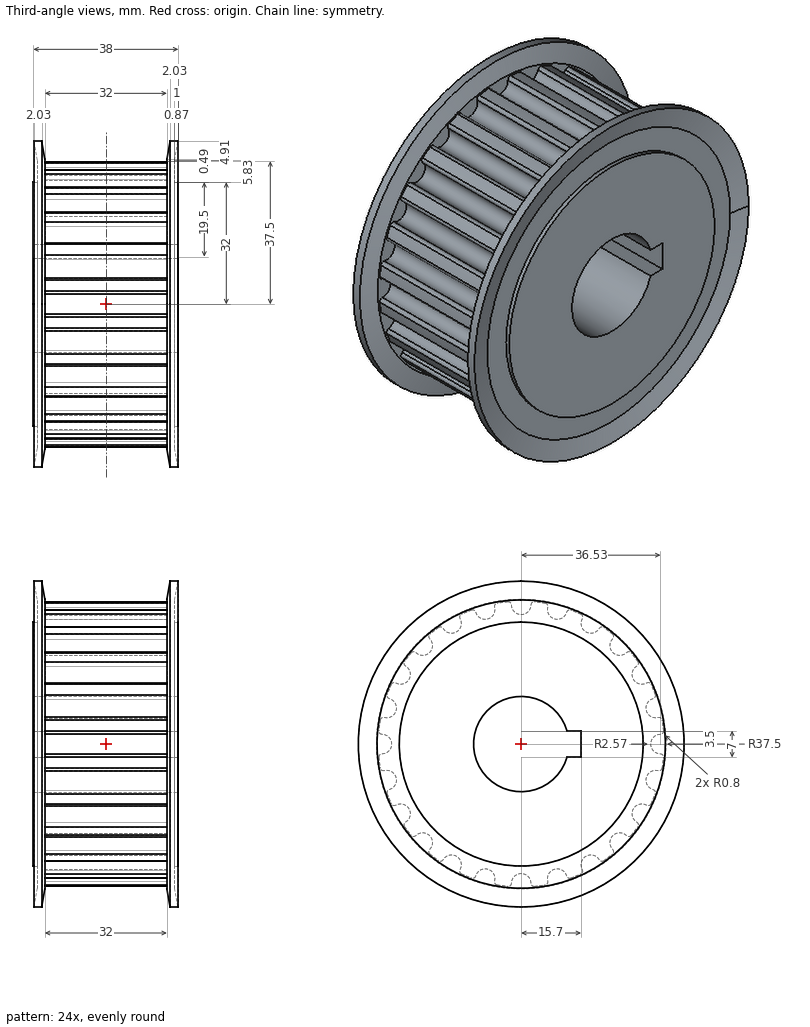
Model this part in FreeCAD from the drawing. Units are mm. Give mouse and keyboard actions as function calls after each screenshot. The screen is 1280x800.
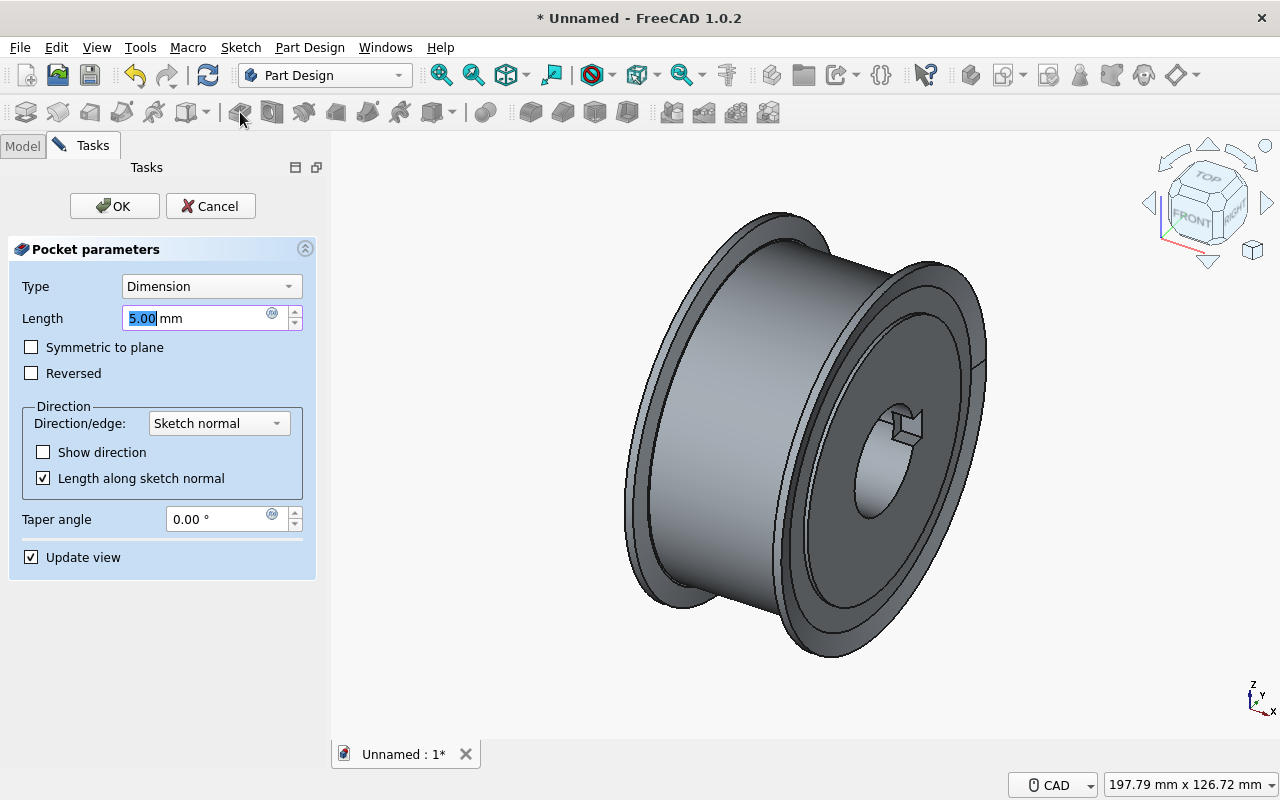
click(212, 286)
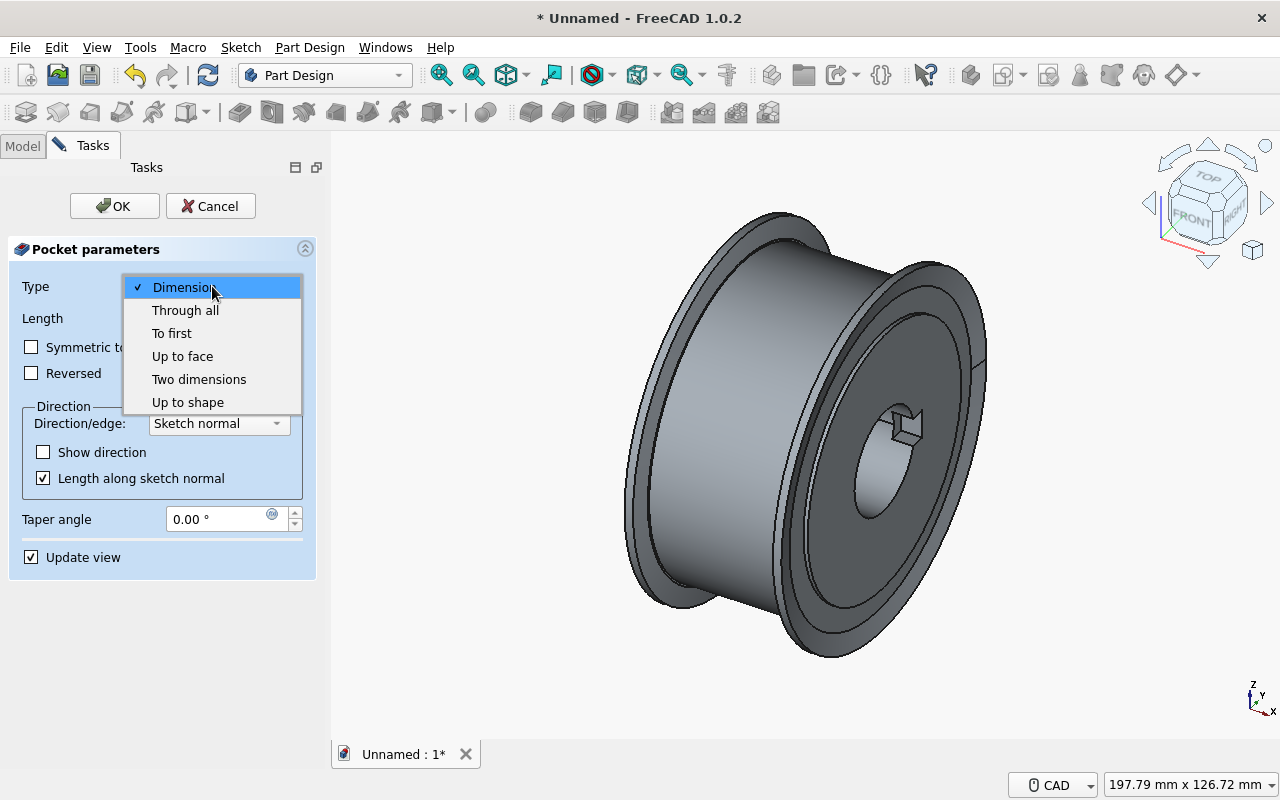
click(212, 310)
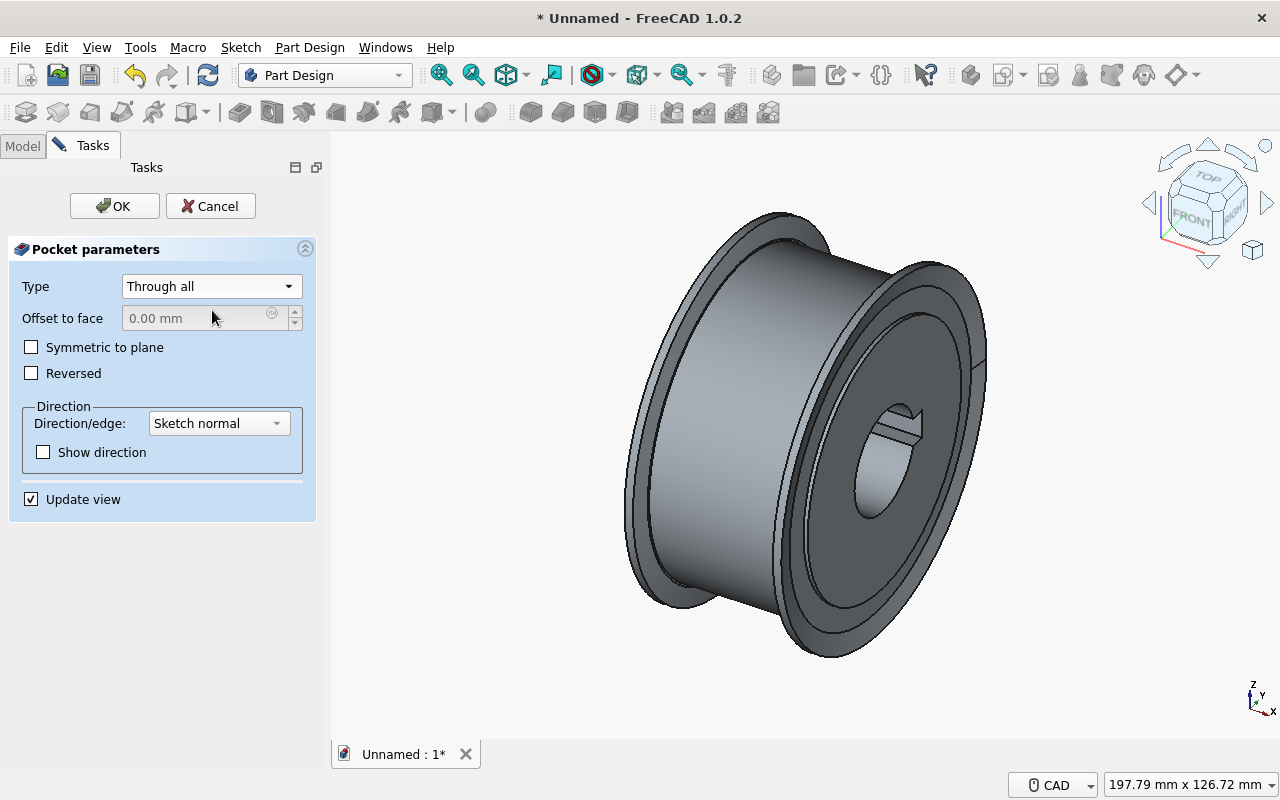
click(115, 206)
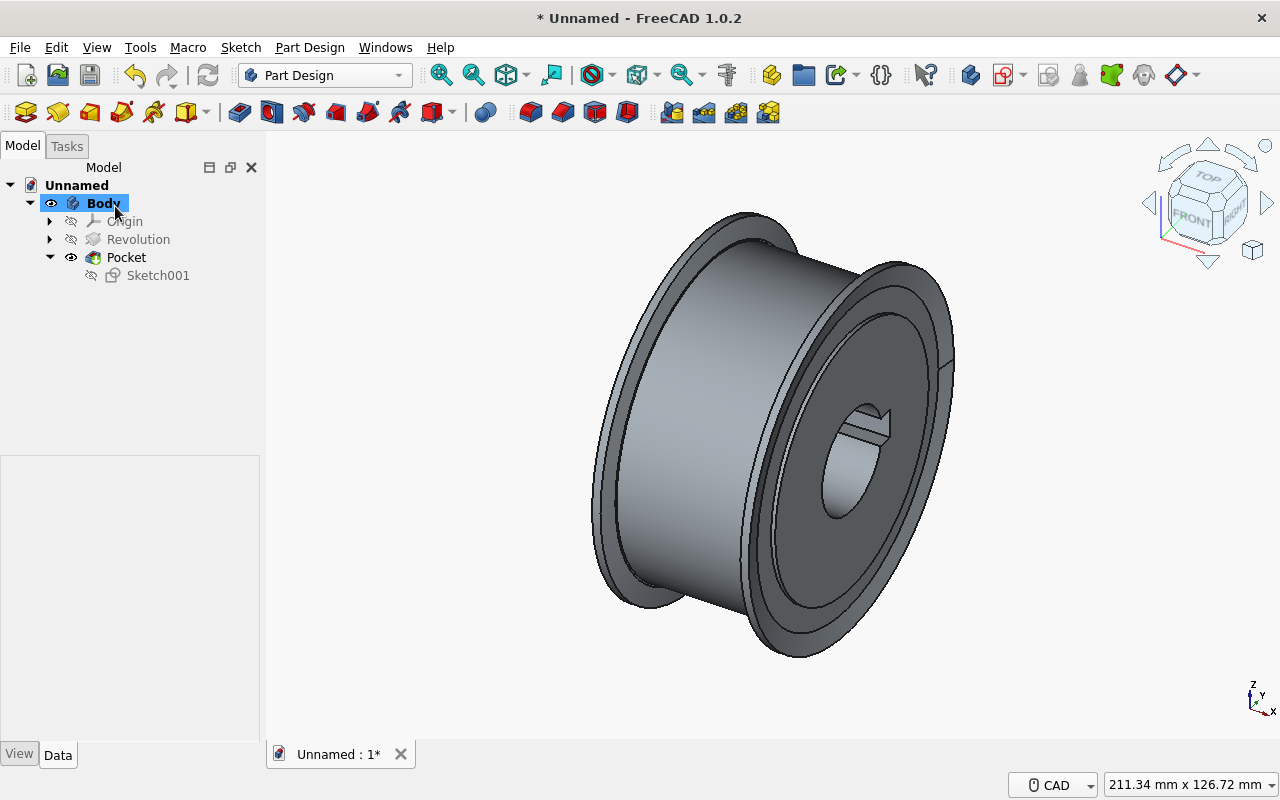
click(50, 221)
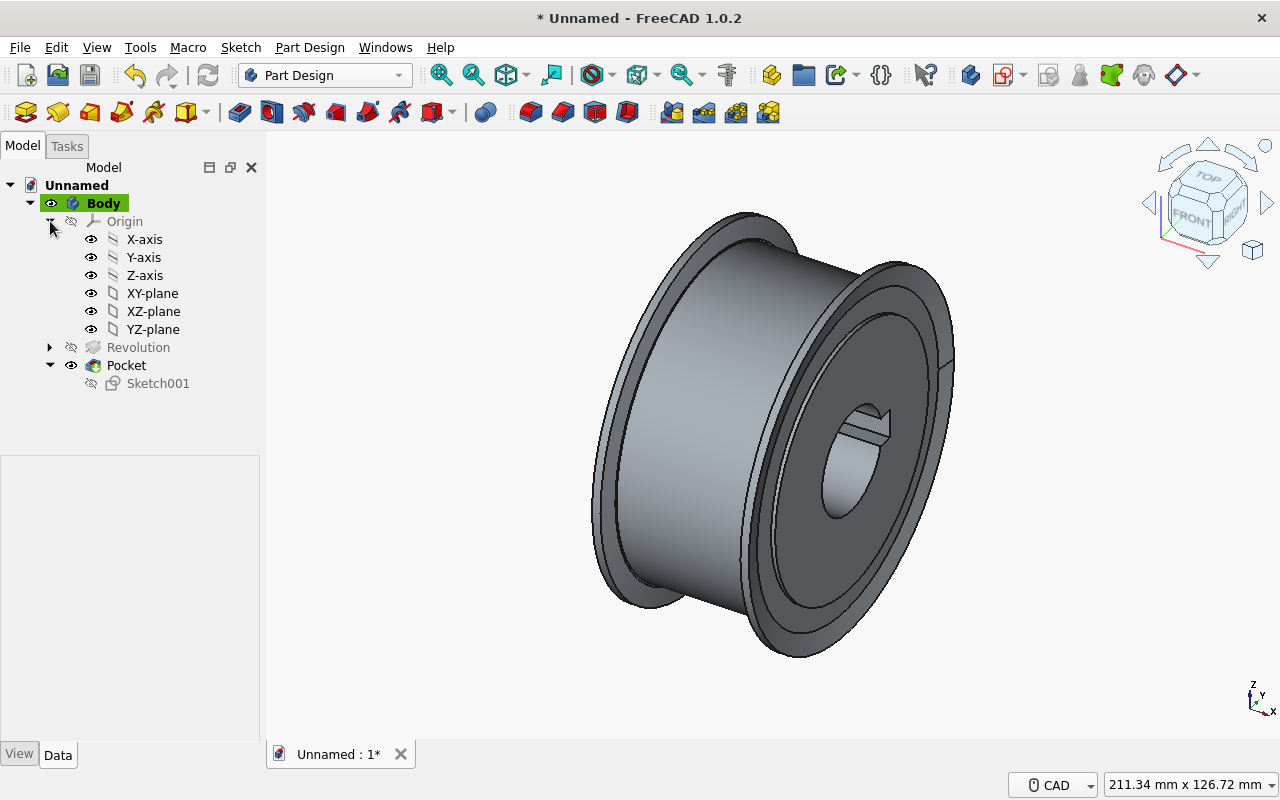
click(136, 329)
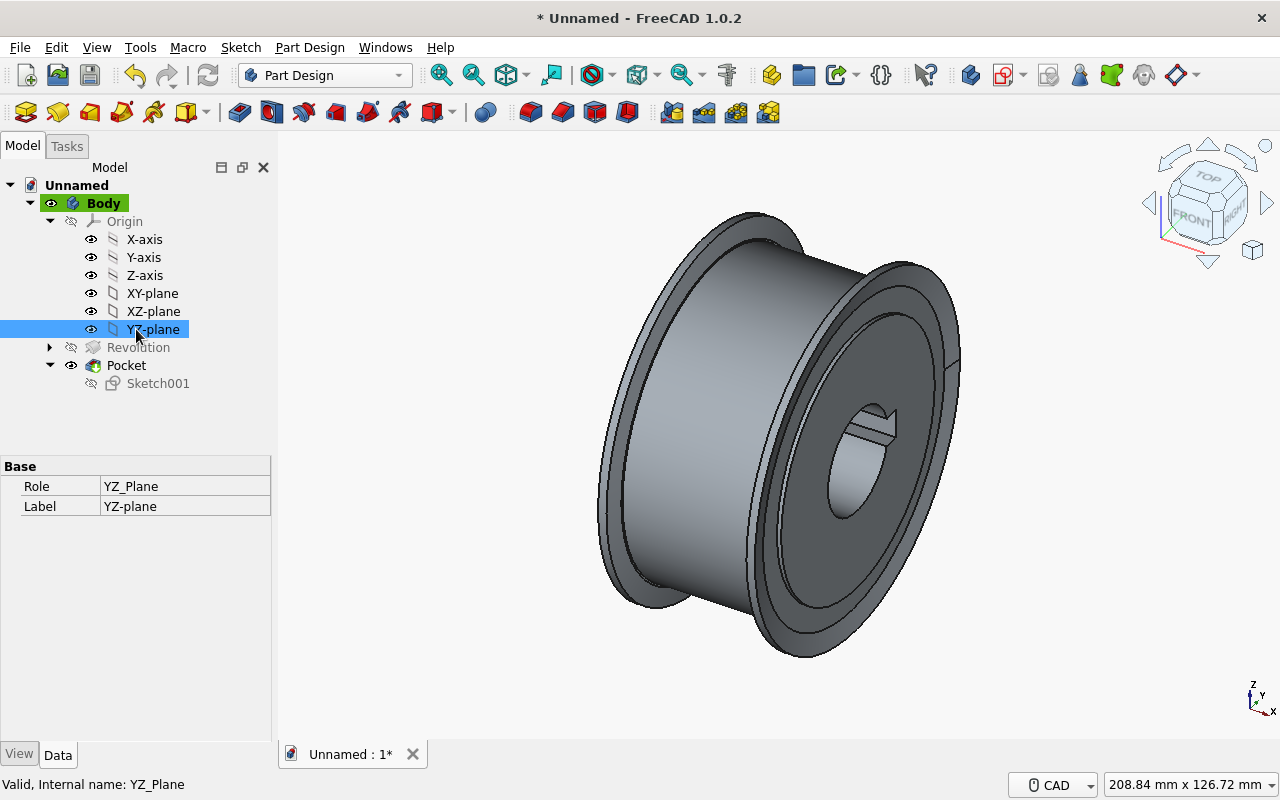
click(1176, 76)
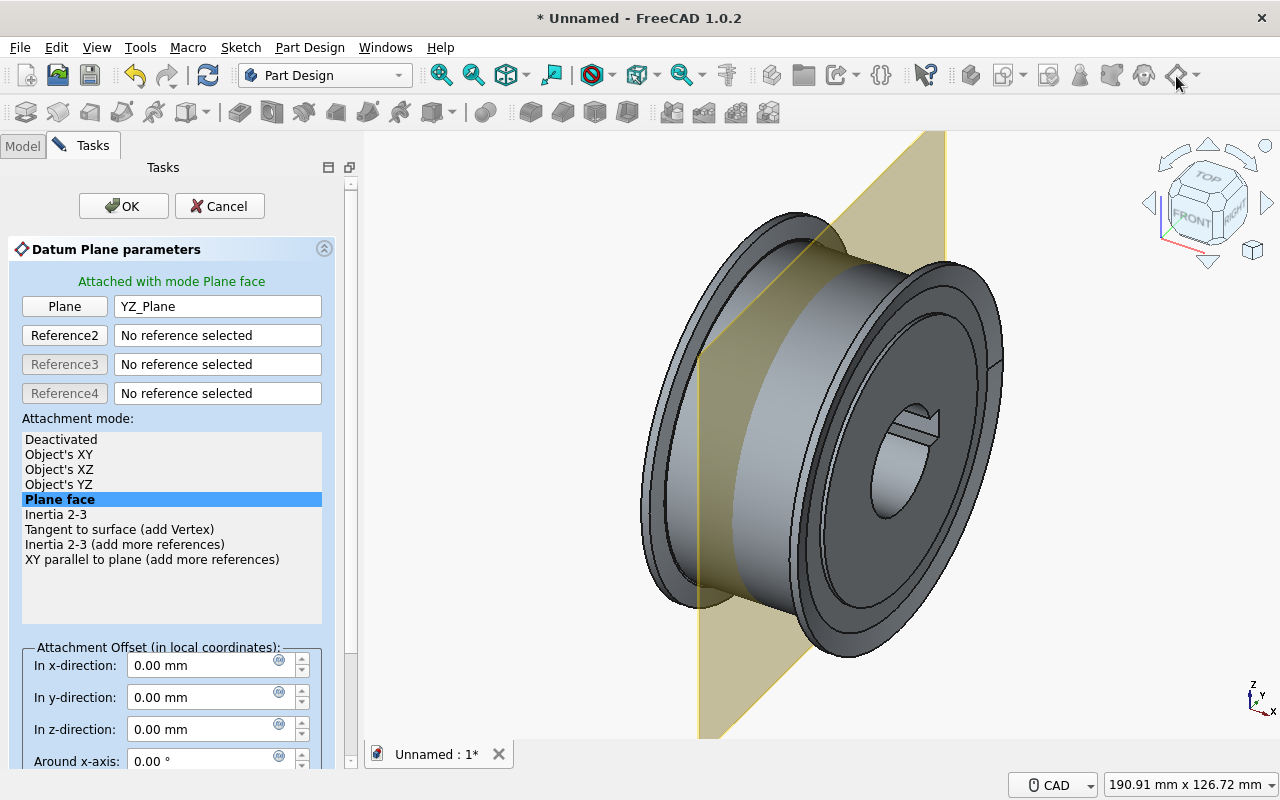
triple_click(210, 729)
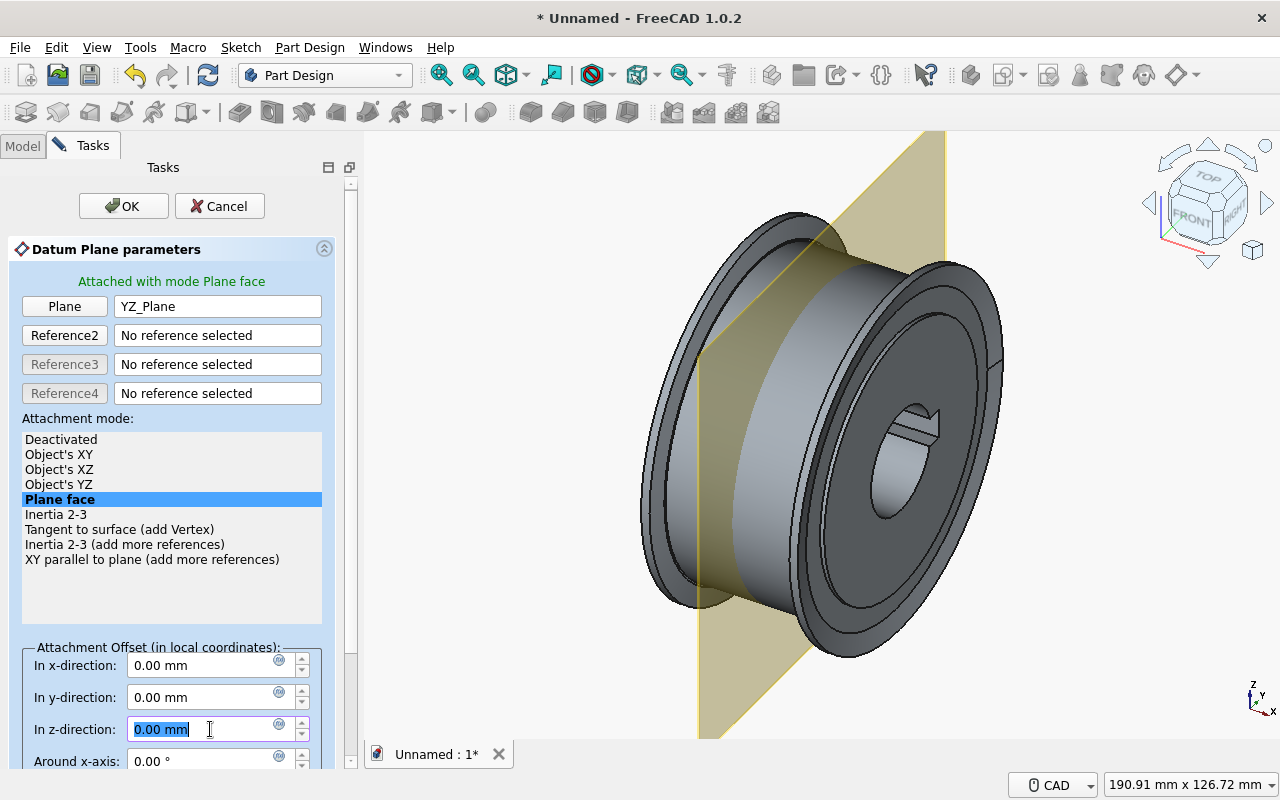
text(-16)
key(Tab)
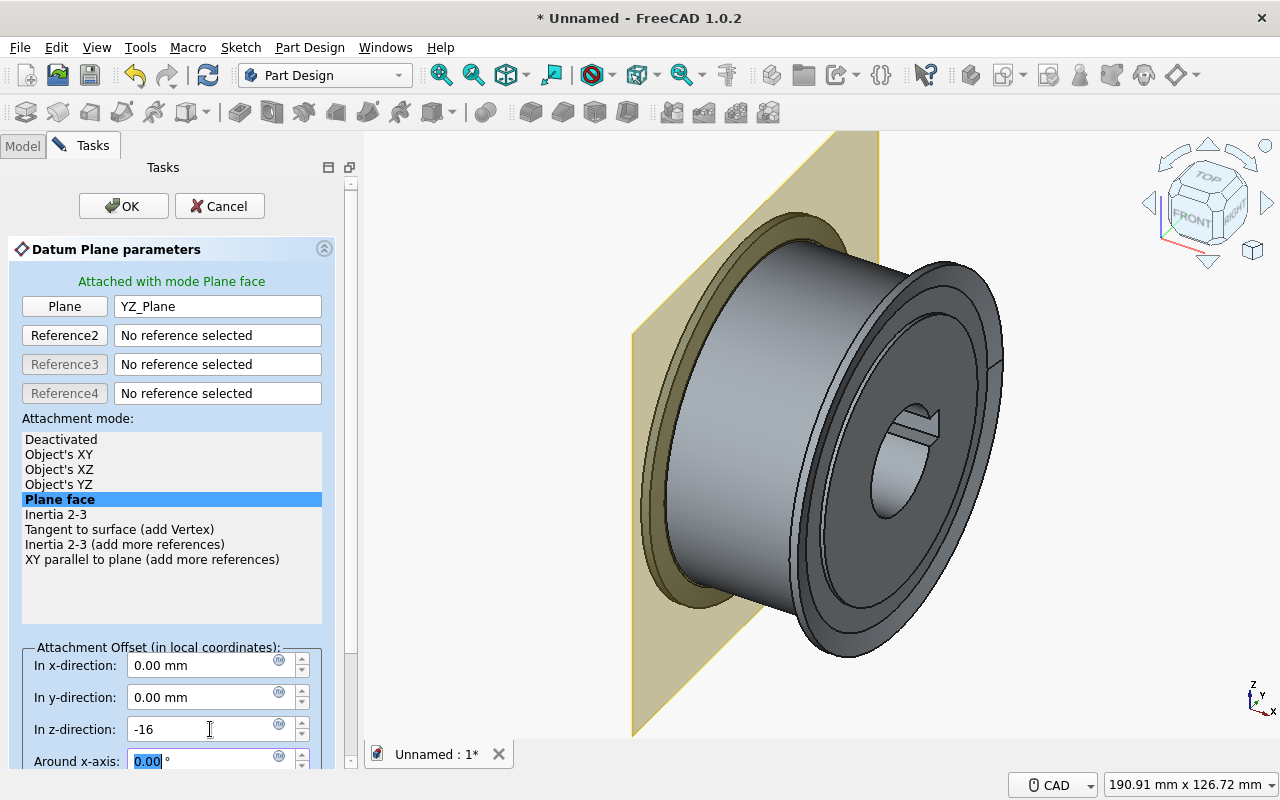
click(124, 206)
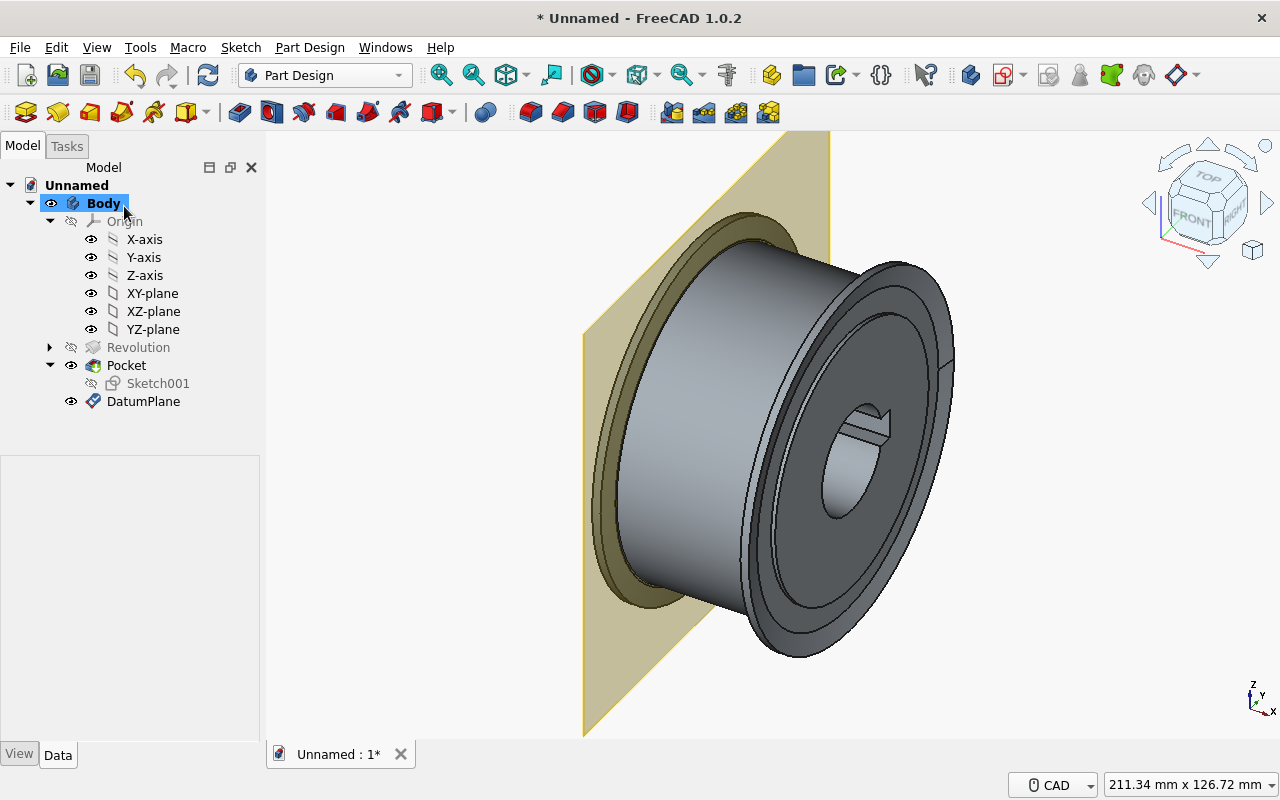
click(116, 401)